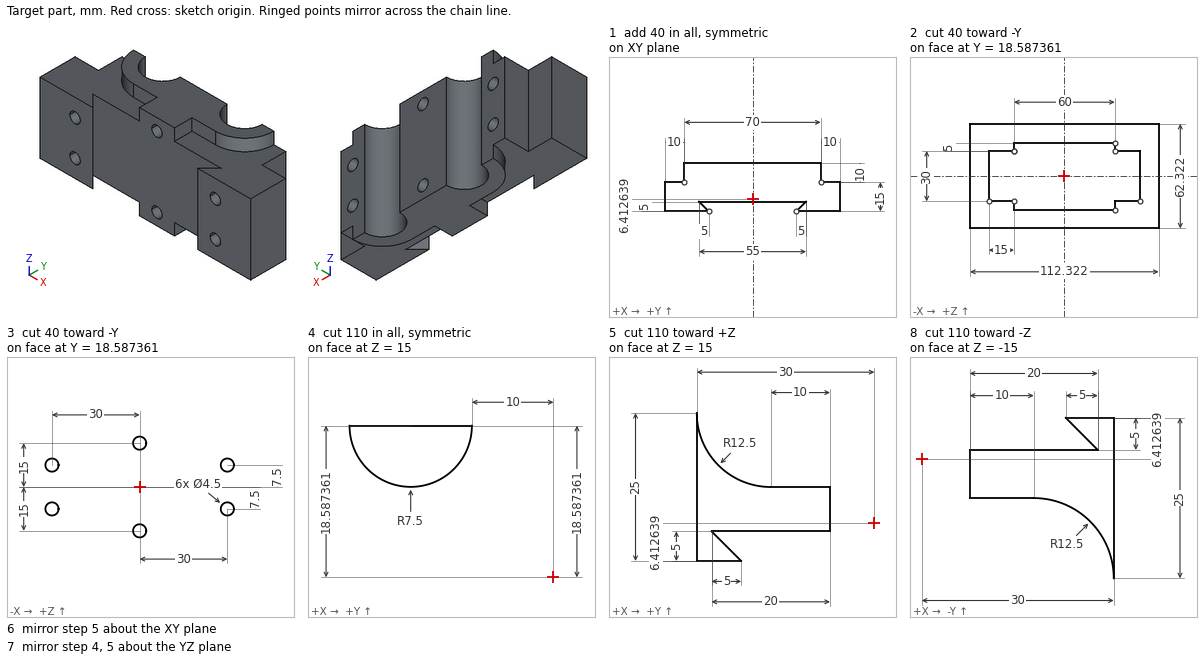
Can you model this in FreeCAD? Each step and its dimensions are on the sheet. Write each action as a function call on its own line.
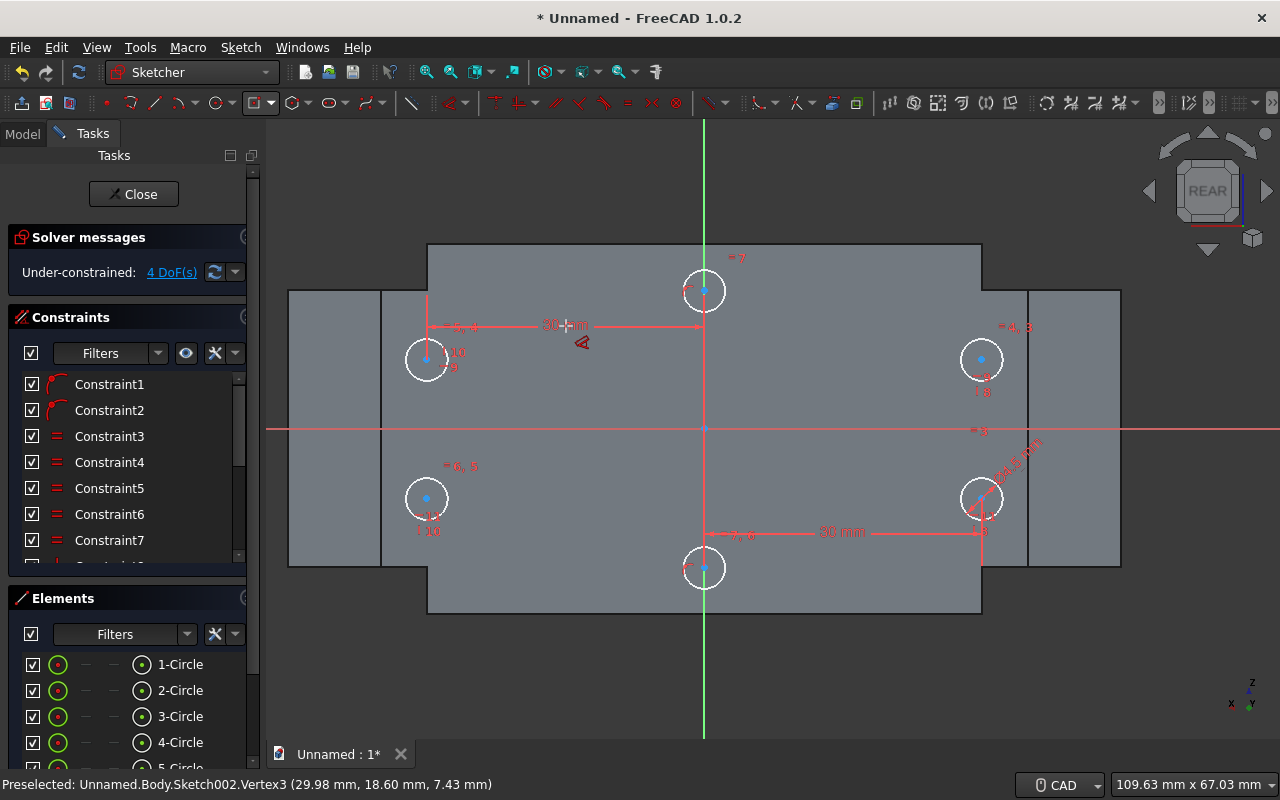
click(704, 568)
click(738, 498)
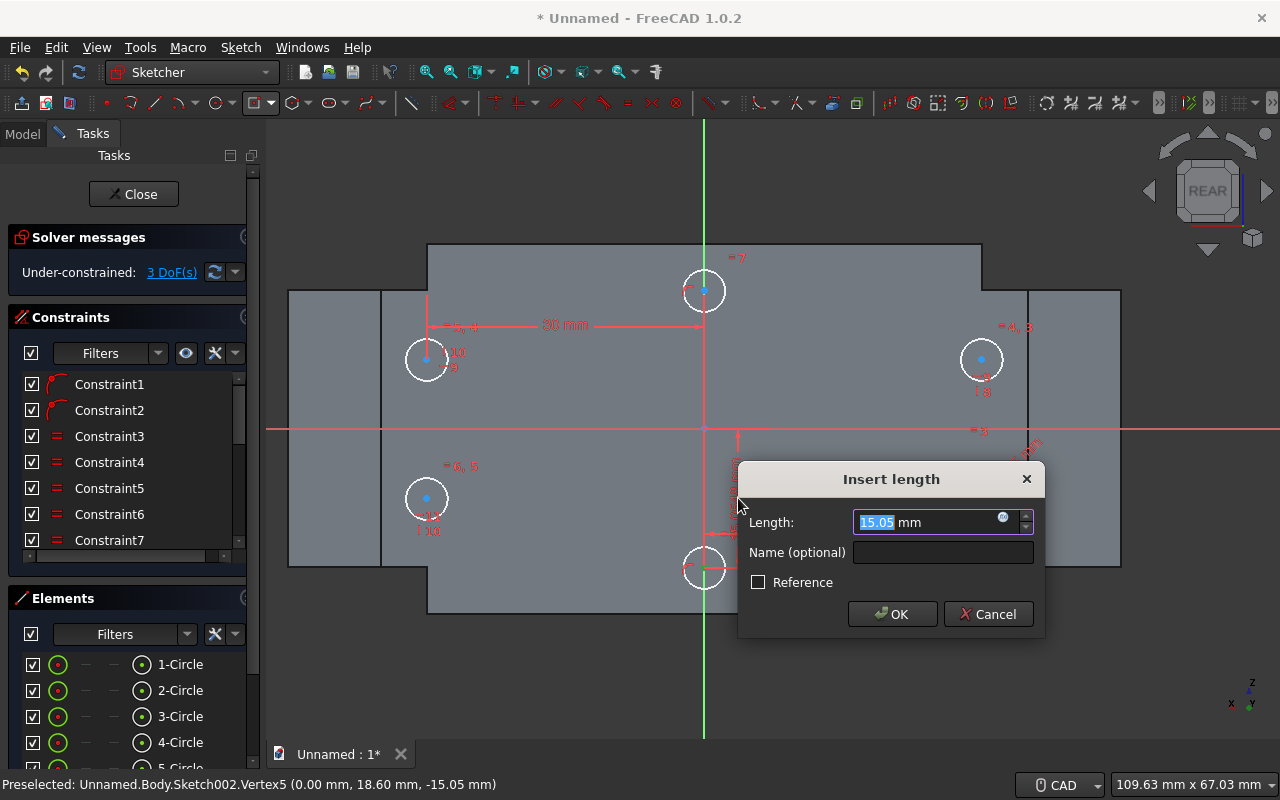
text(15)
key(Return)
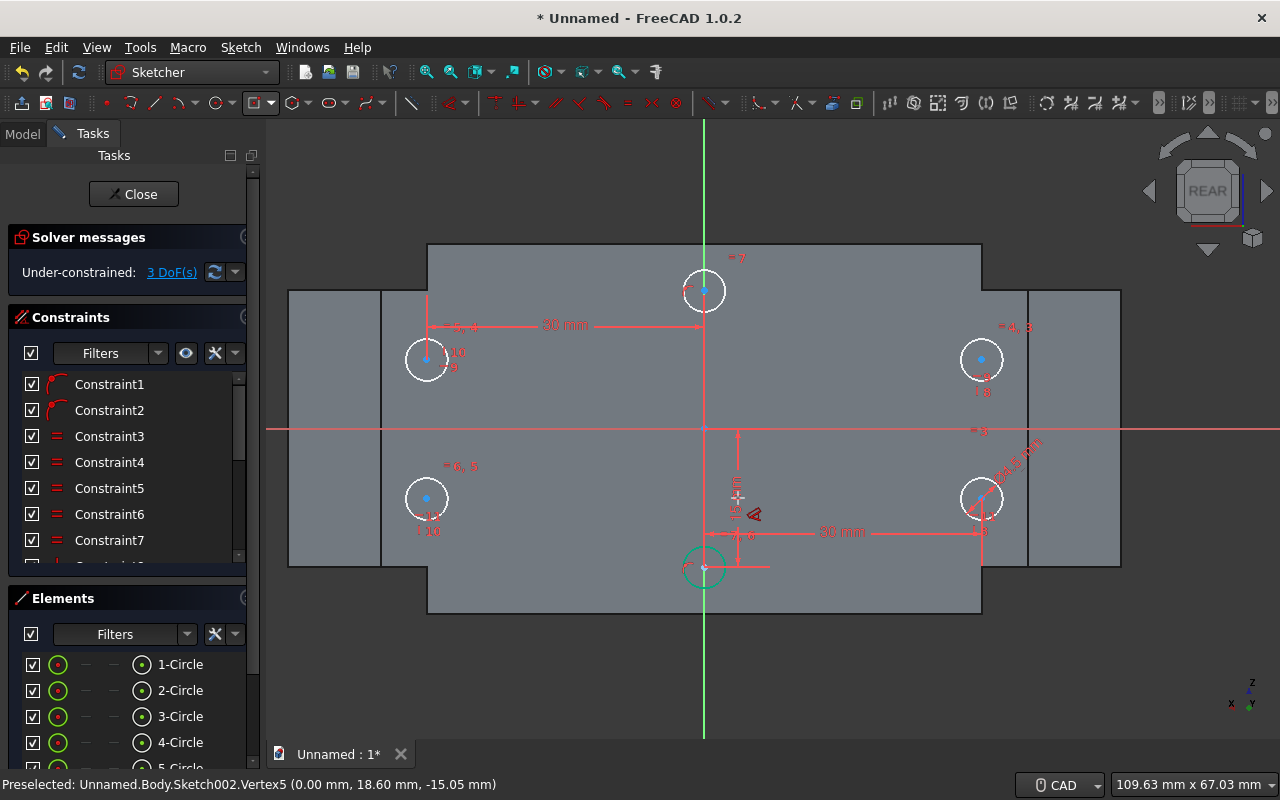
click(704, 291)
click(738, 360)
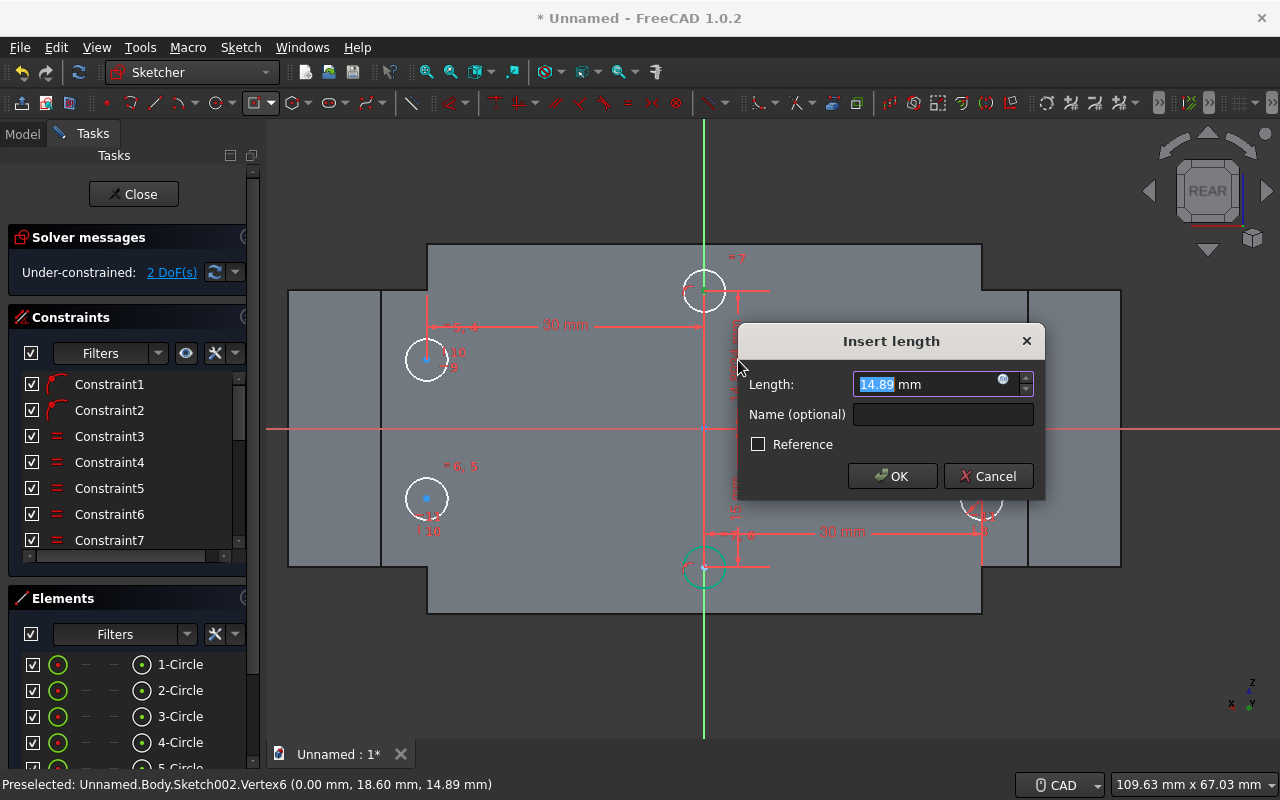
text(15)
key(Return)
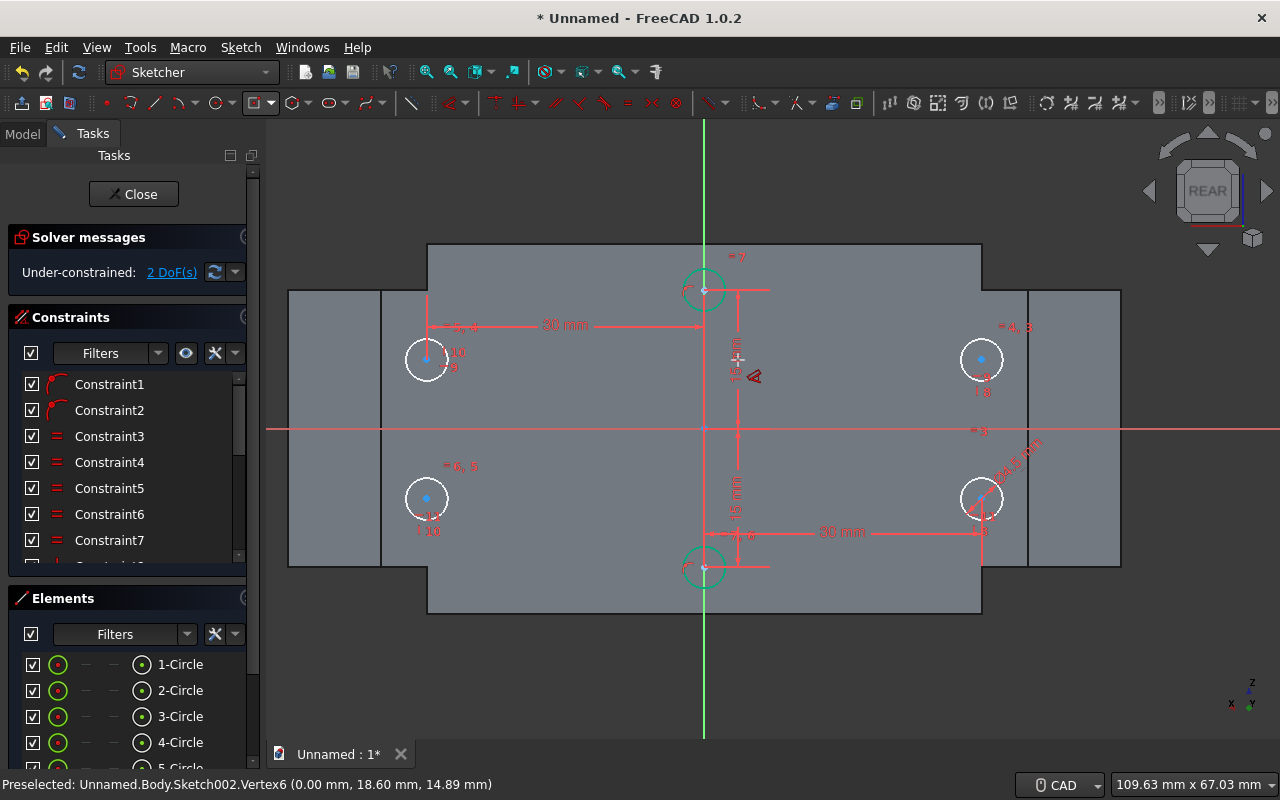
click(982, 499)
click(1016, 488)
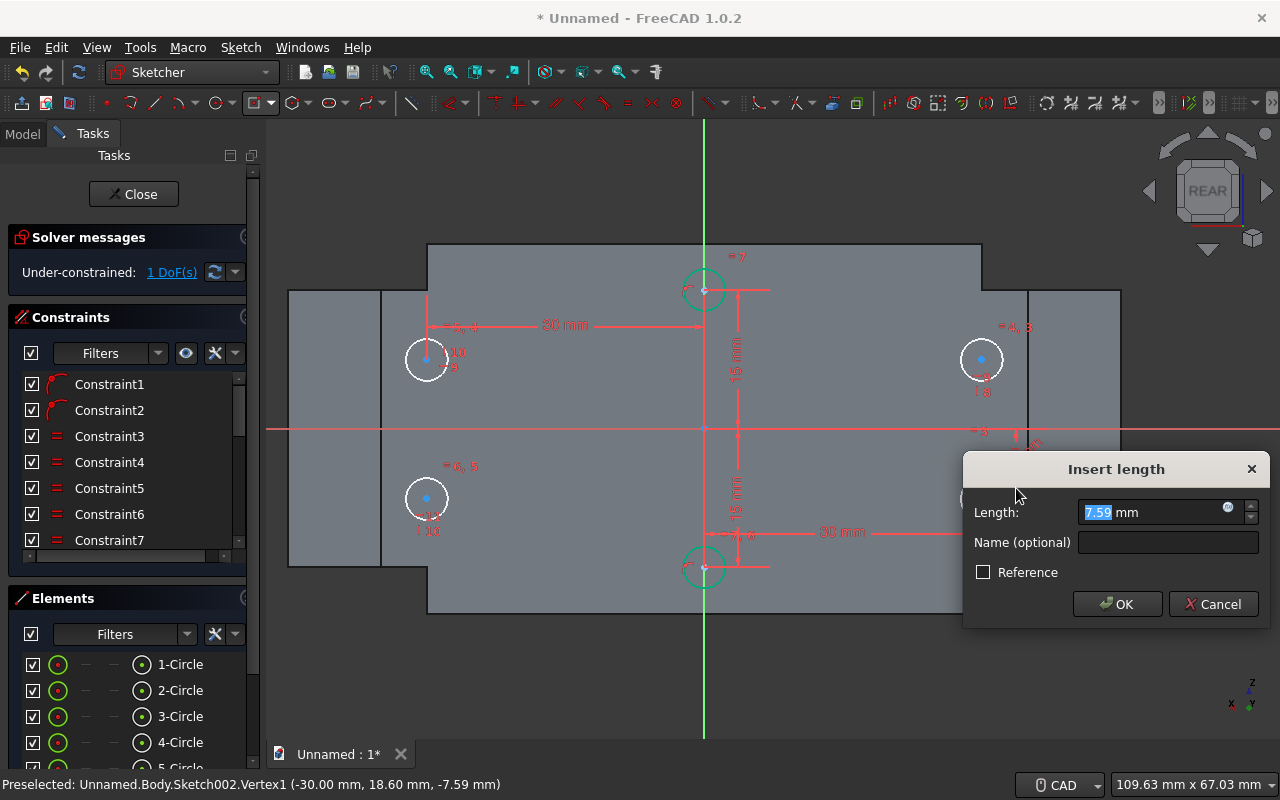
text(7.5)
key(Return)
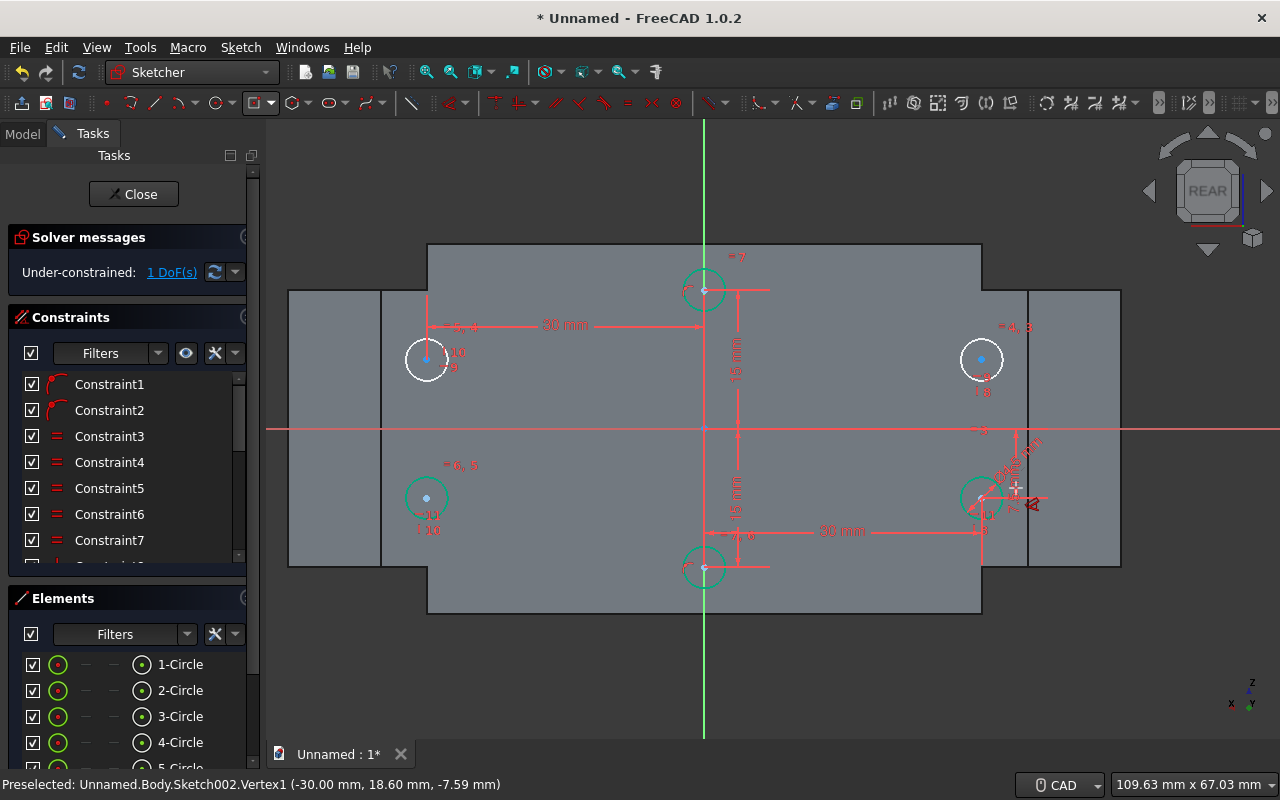
click(982, 360)
click(1016, 394)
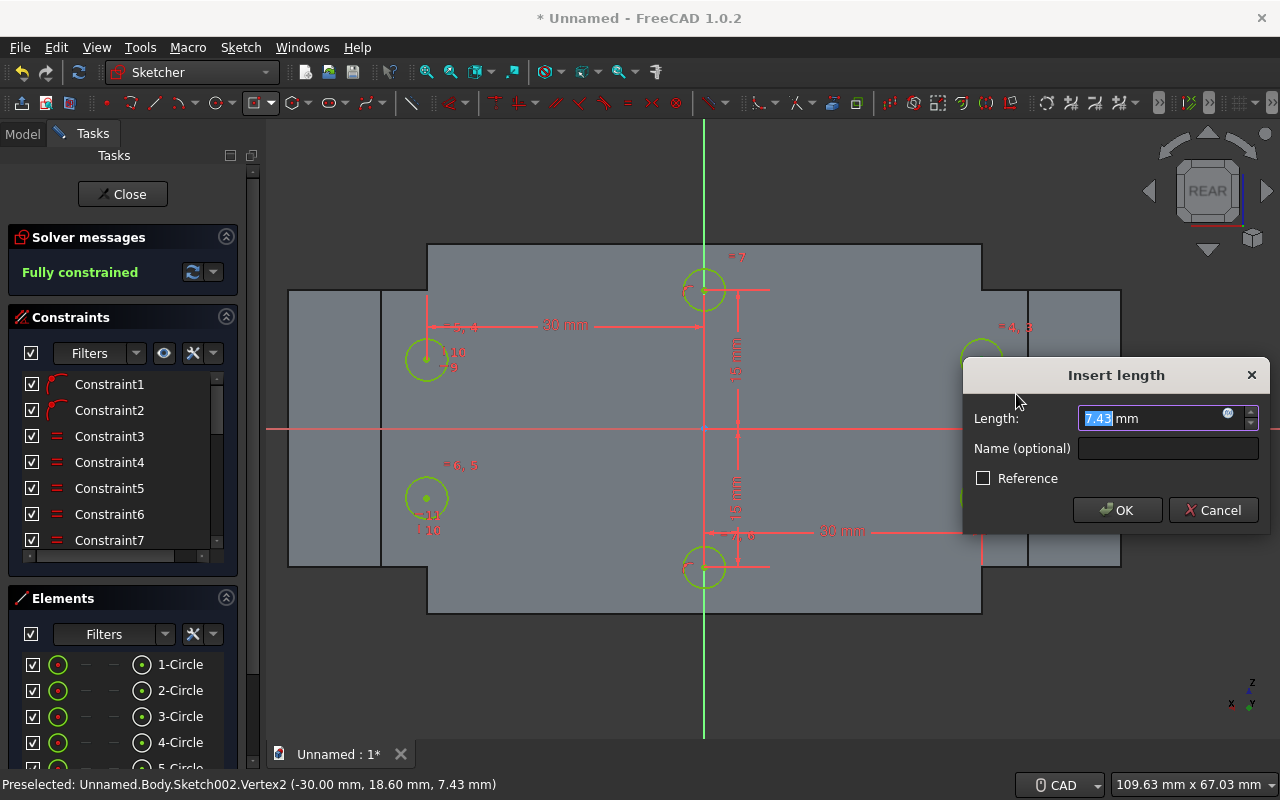
text(7.5)
key(Return)
key(Escape)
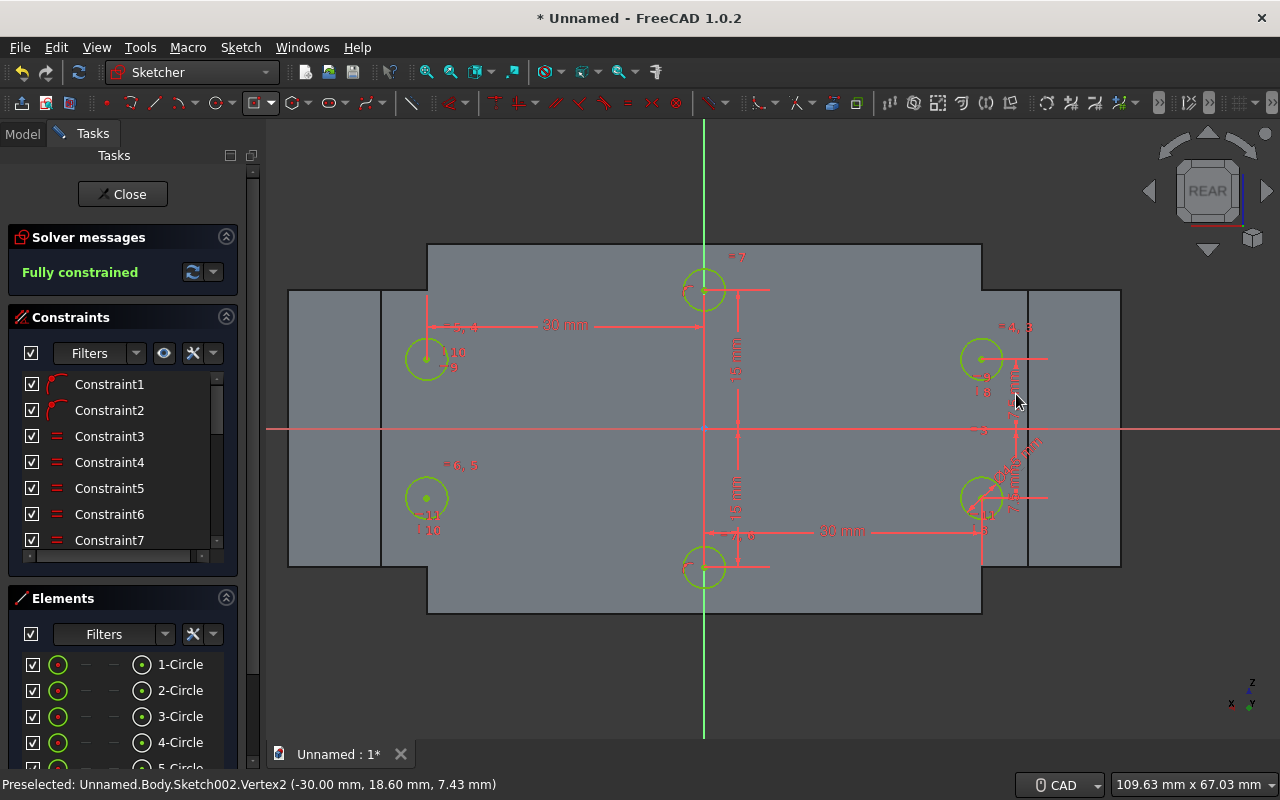
click(123, 194)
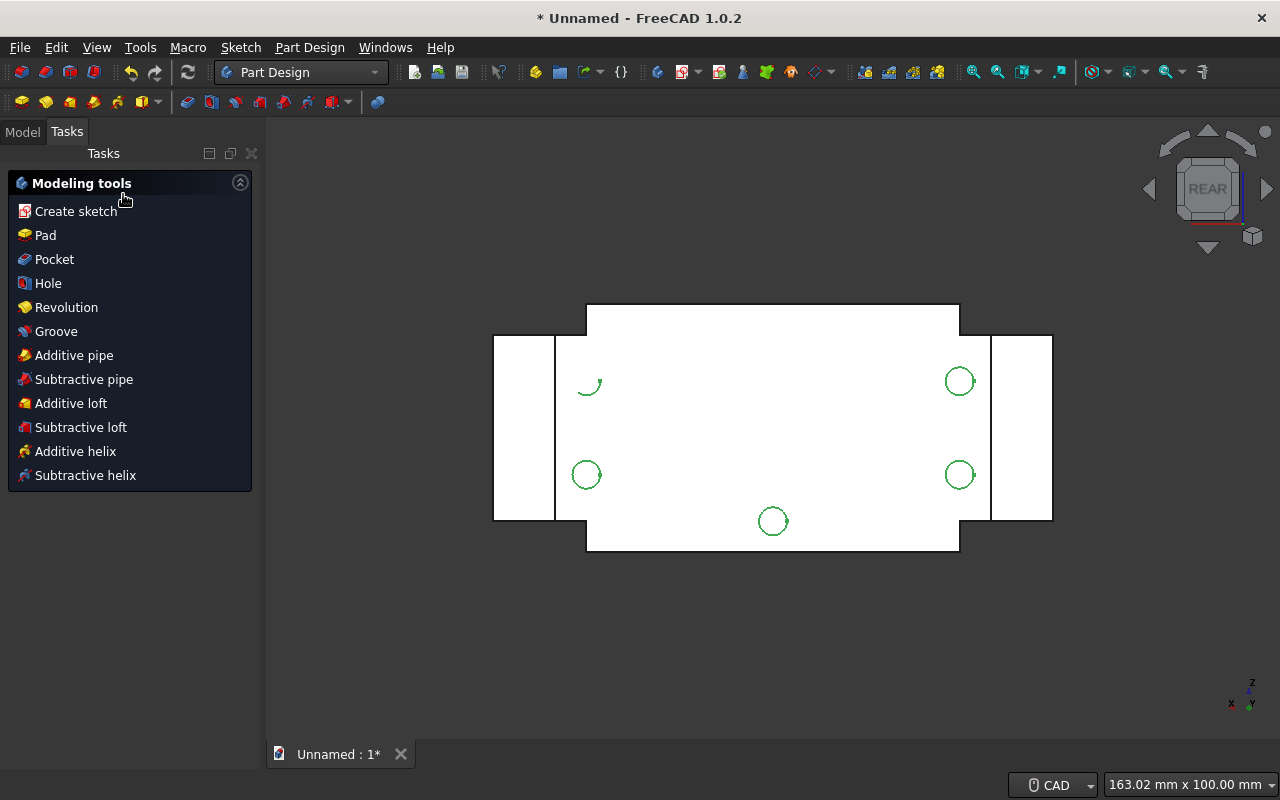
click(188, 102)